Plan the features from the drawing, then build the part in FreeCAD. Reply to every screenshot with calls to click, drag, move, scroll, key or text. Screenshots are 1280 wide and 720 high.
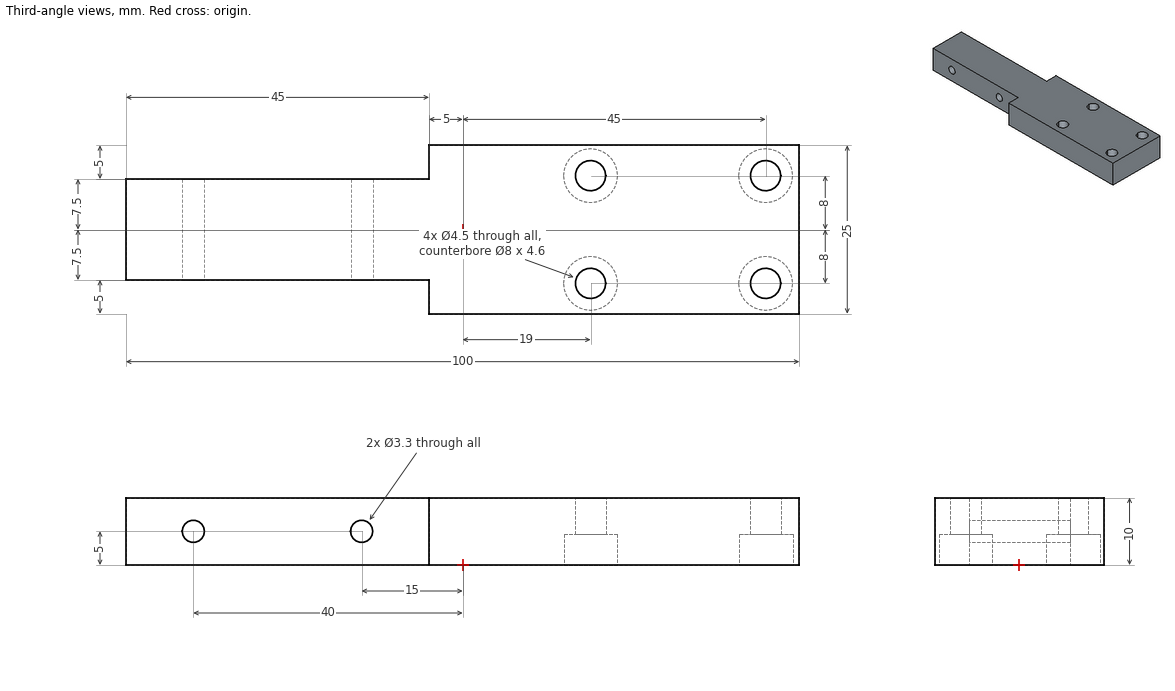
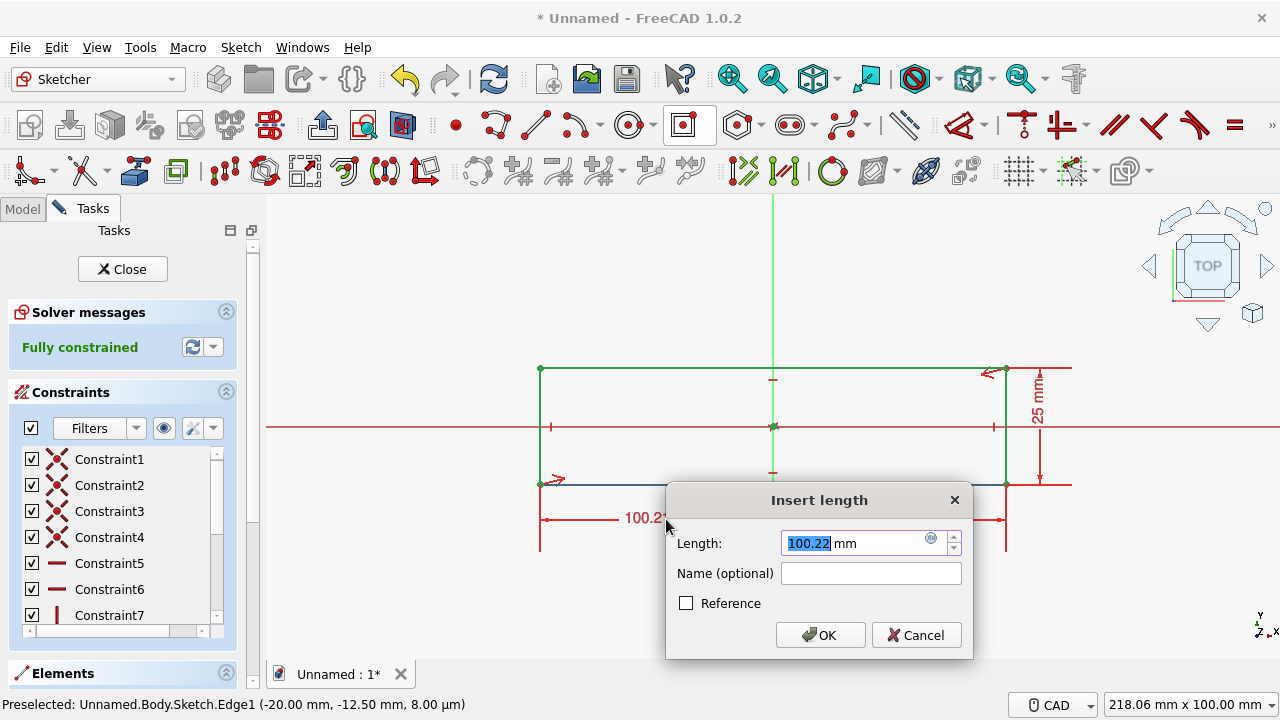
text(100)
key(Return)
key(Escape)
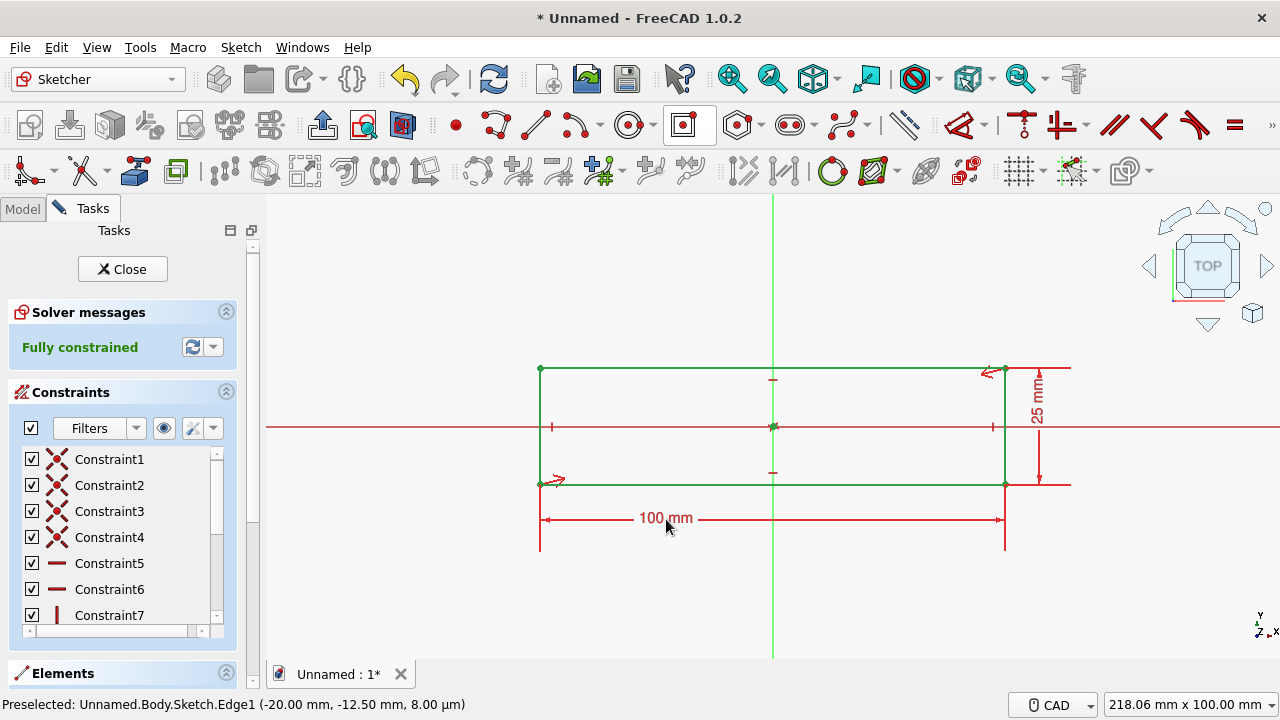
click(123, 269)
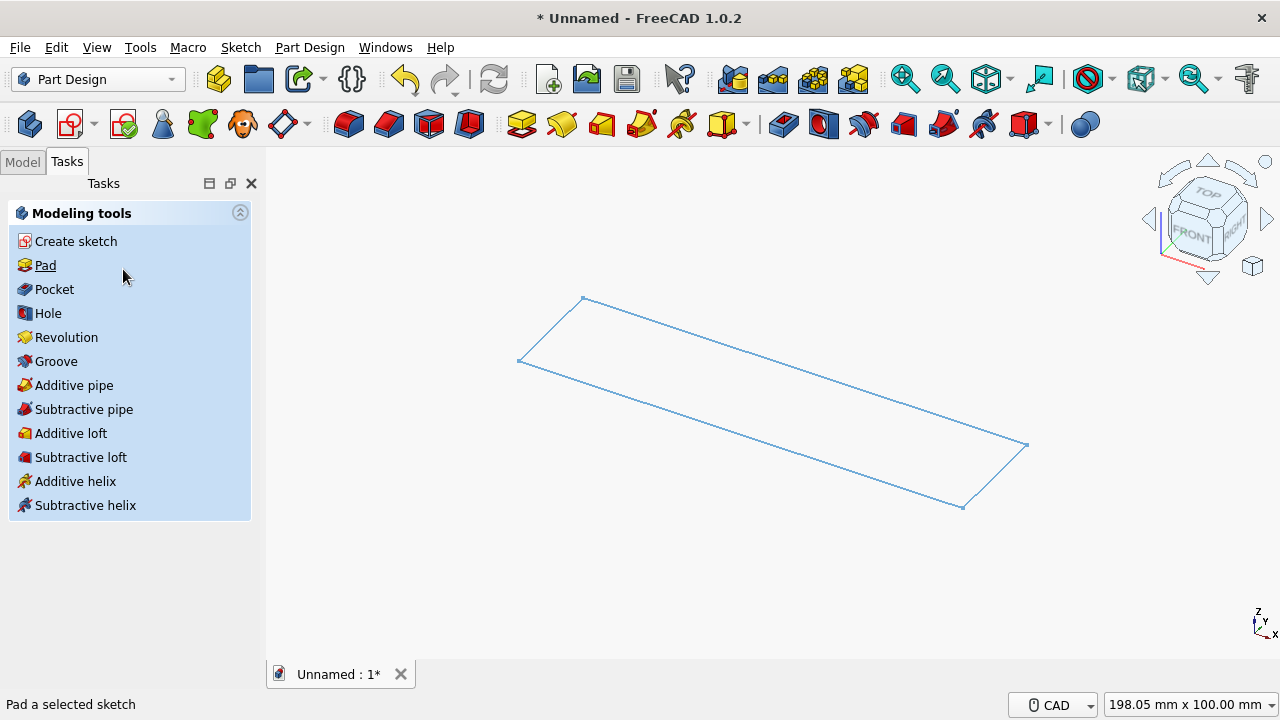
click(522, 124)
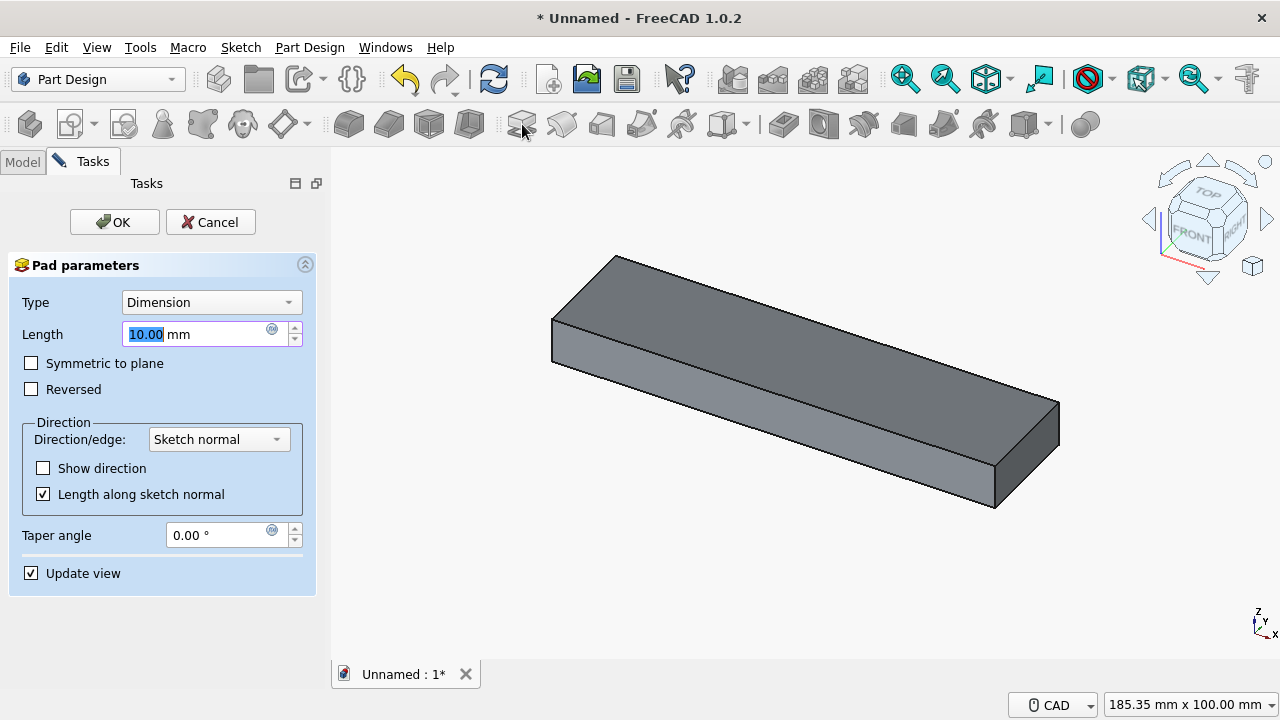
text(10)
key(Tab)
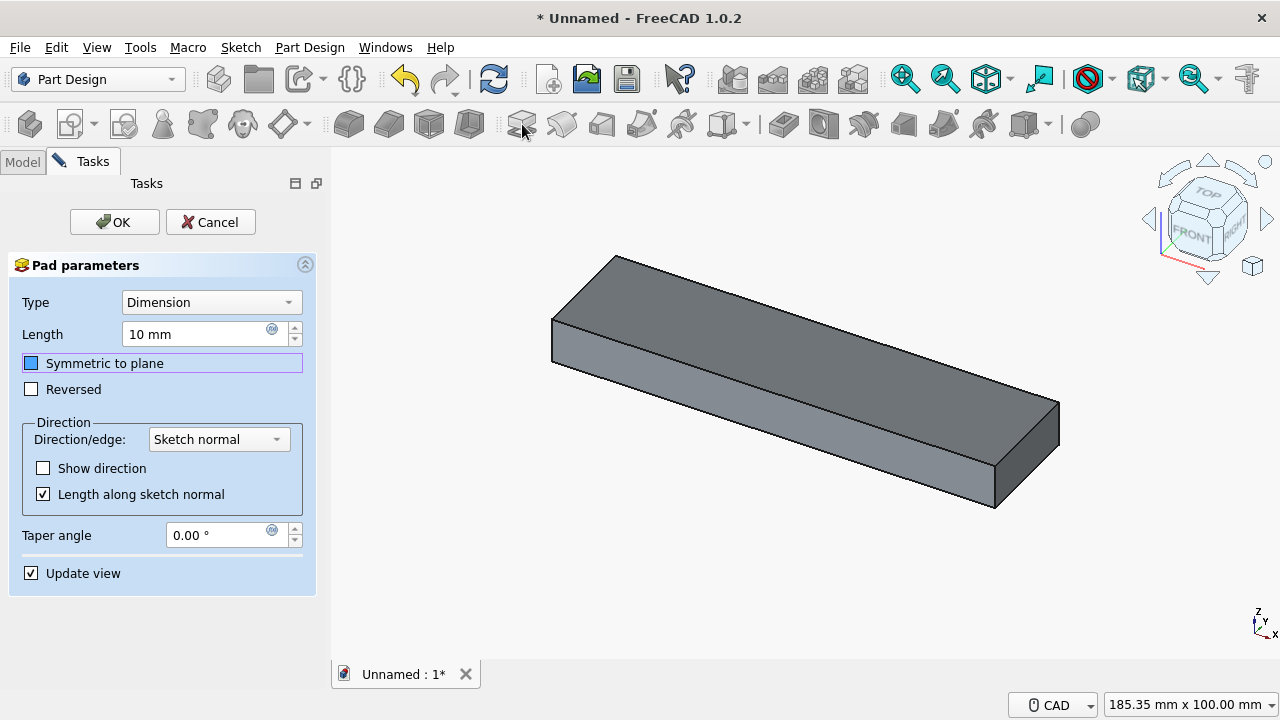
click(115, 222)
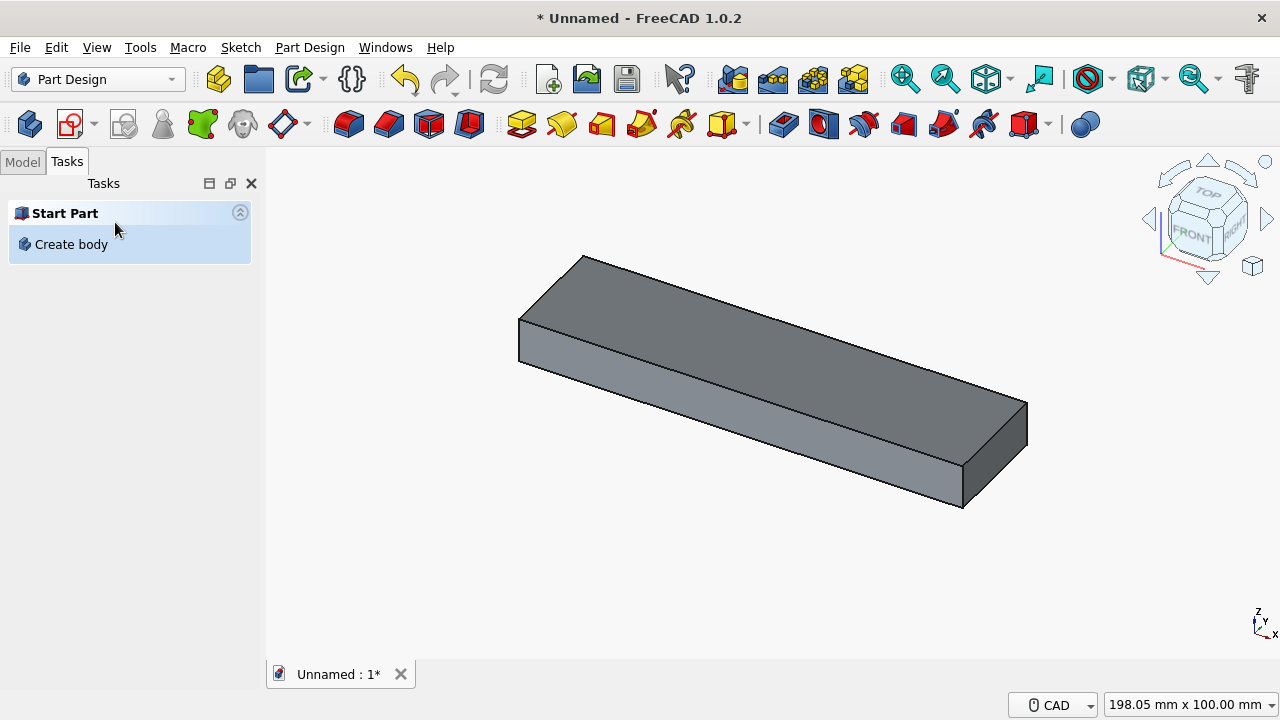
click(70, 124)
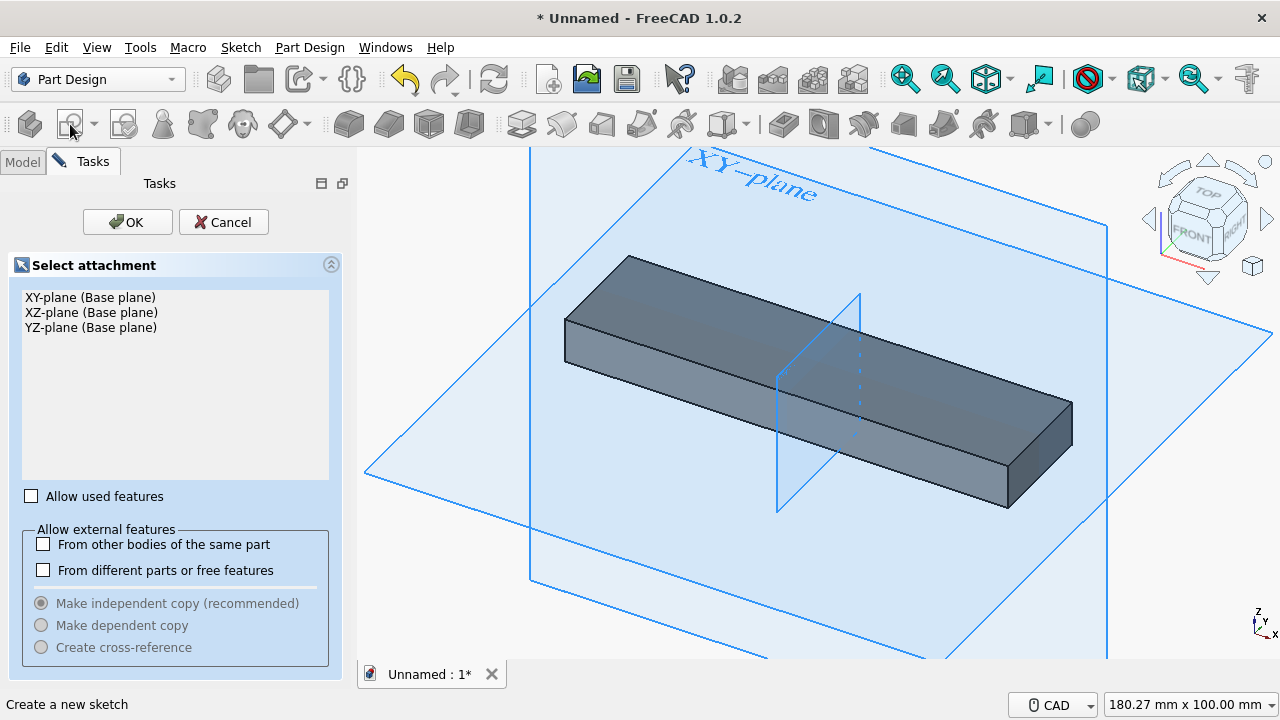
click(82, 298)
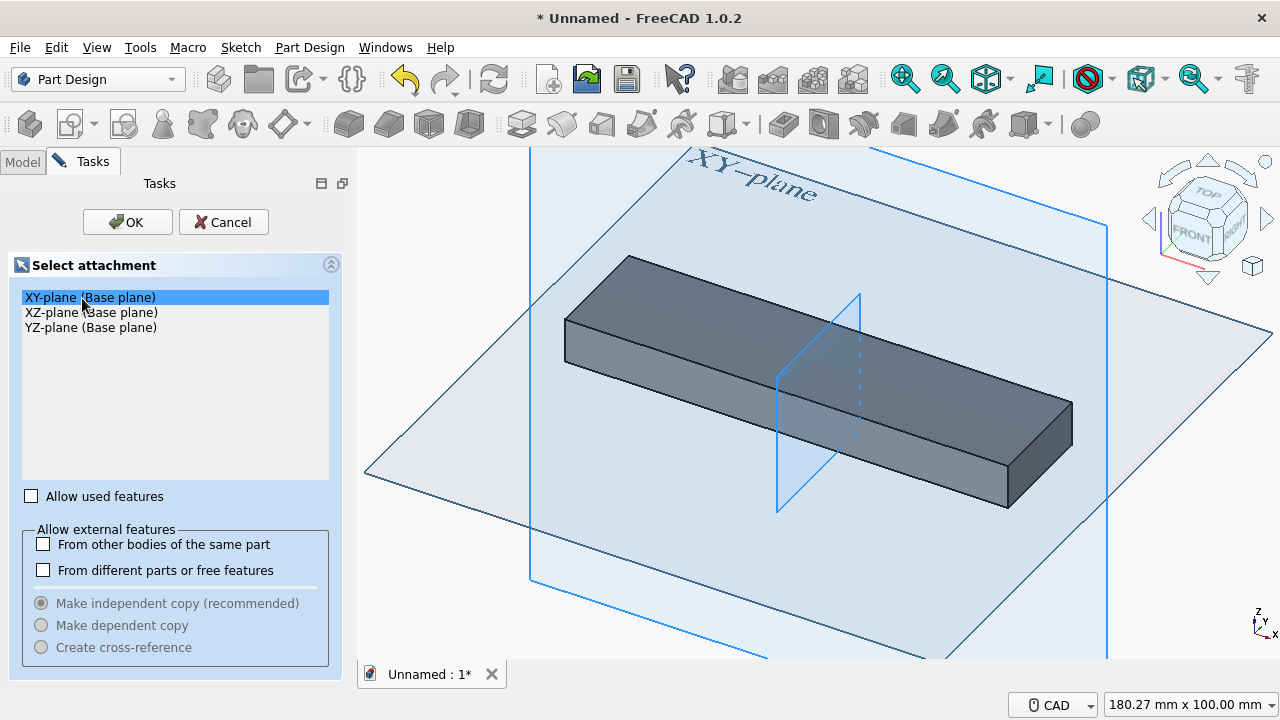
click(128, 222)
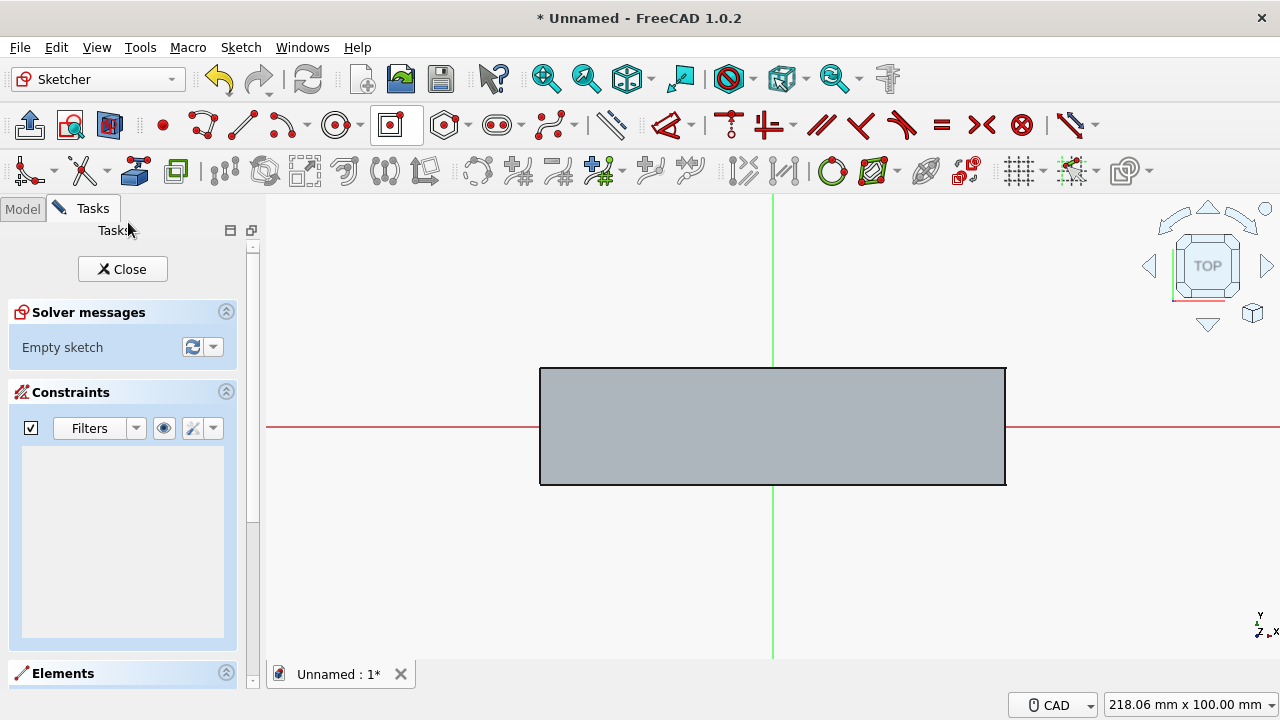
click(110, 126)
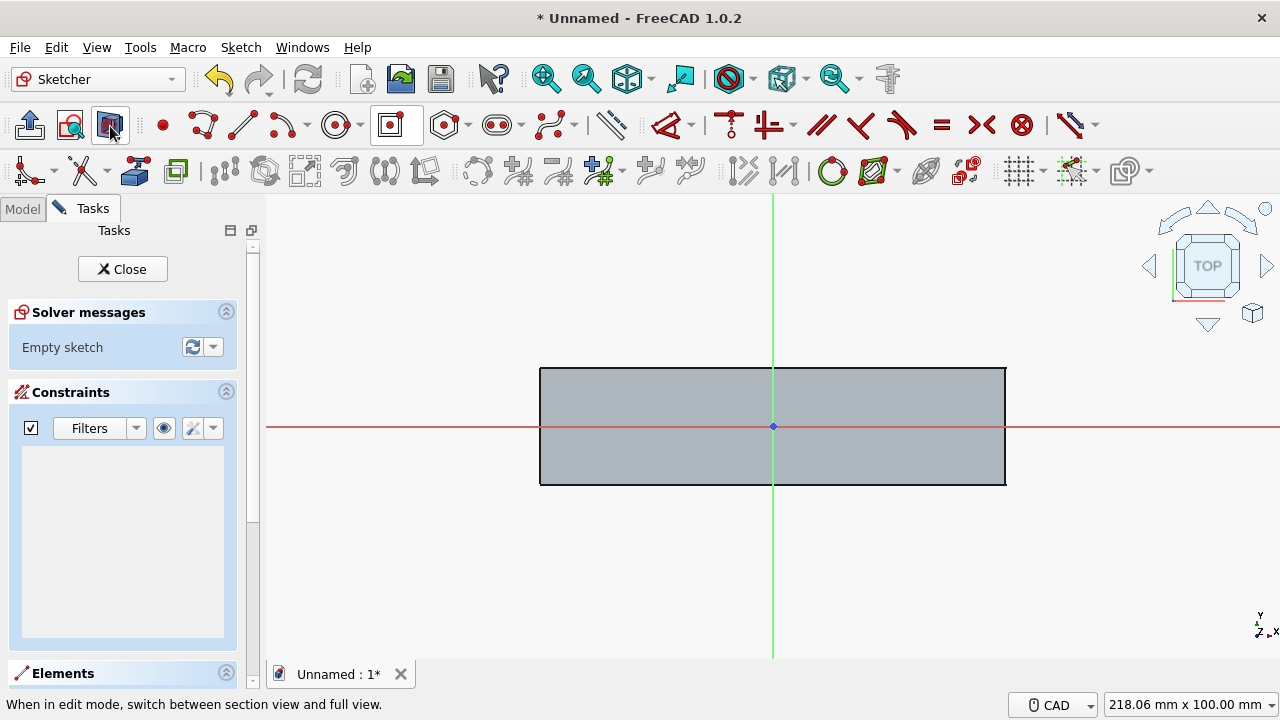
scroll(629, 426, up, 5)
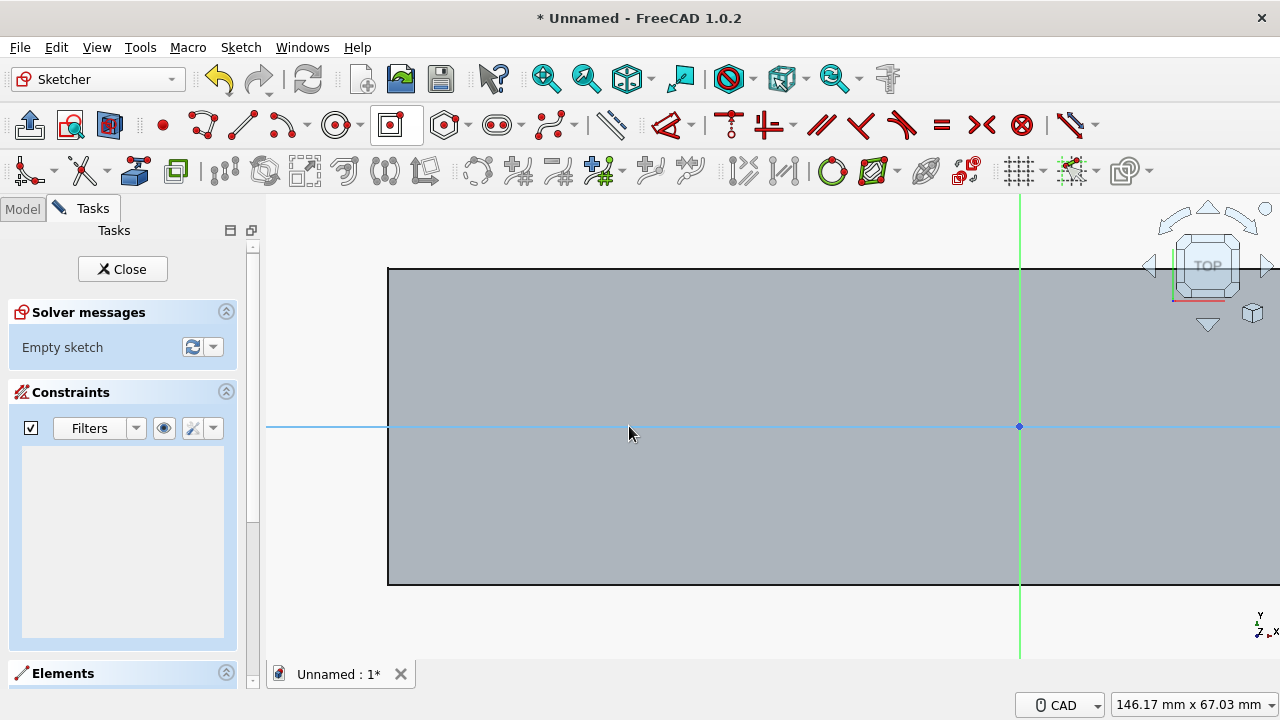
key(g)
key(r)